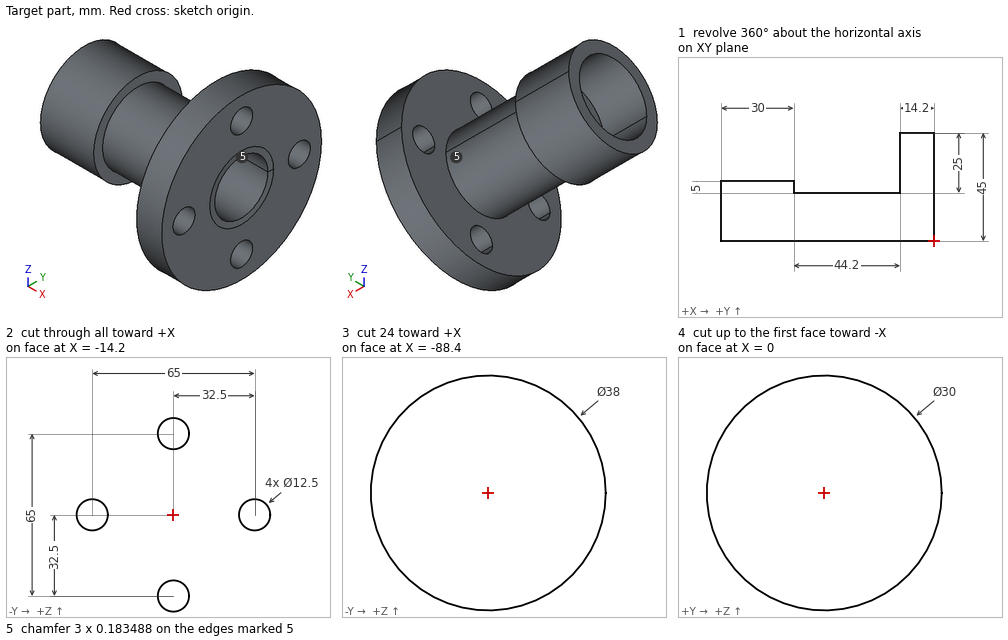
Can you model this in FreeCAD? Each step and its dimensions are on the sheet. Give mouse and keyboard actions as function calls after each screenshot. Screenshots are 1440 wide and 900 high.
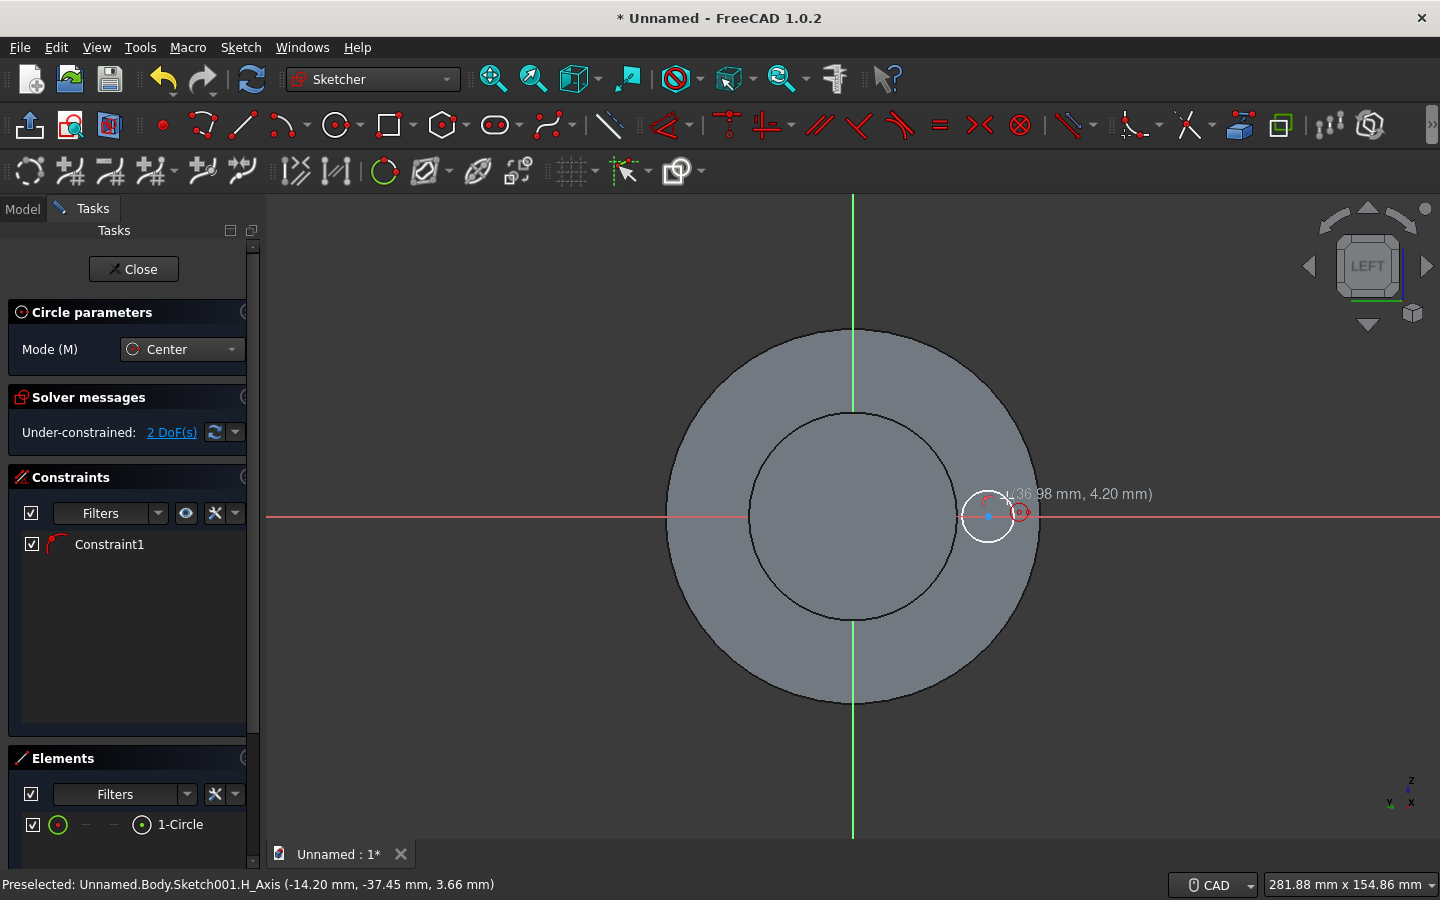
click(853, 652)
click(871, 633)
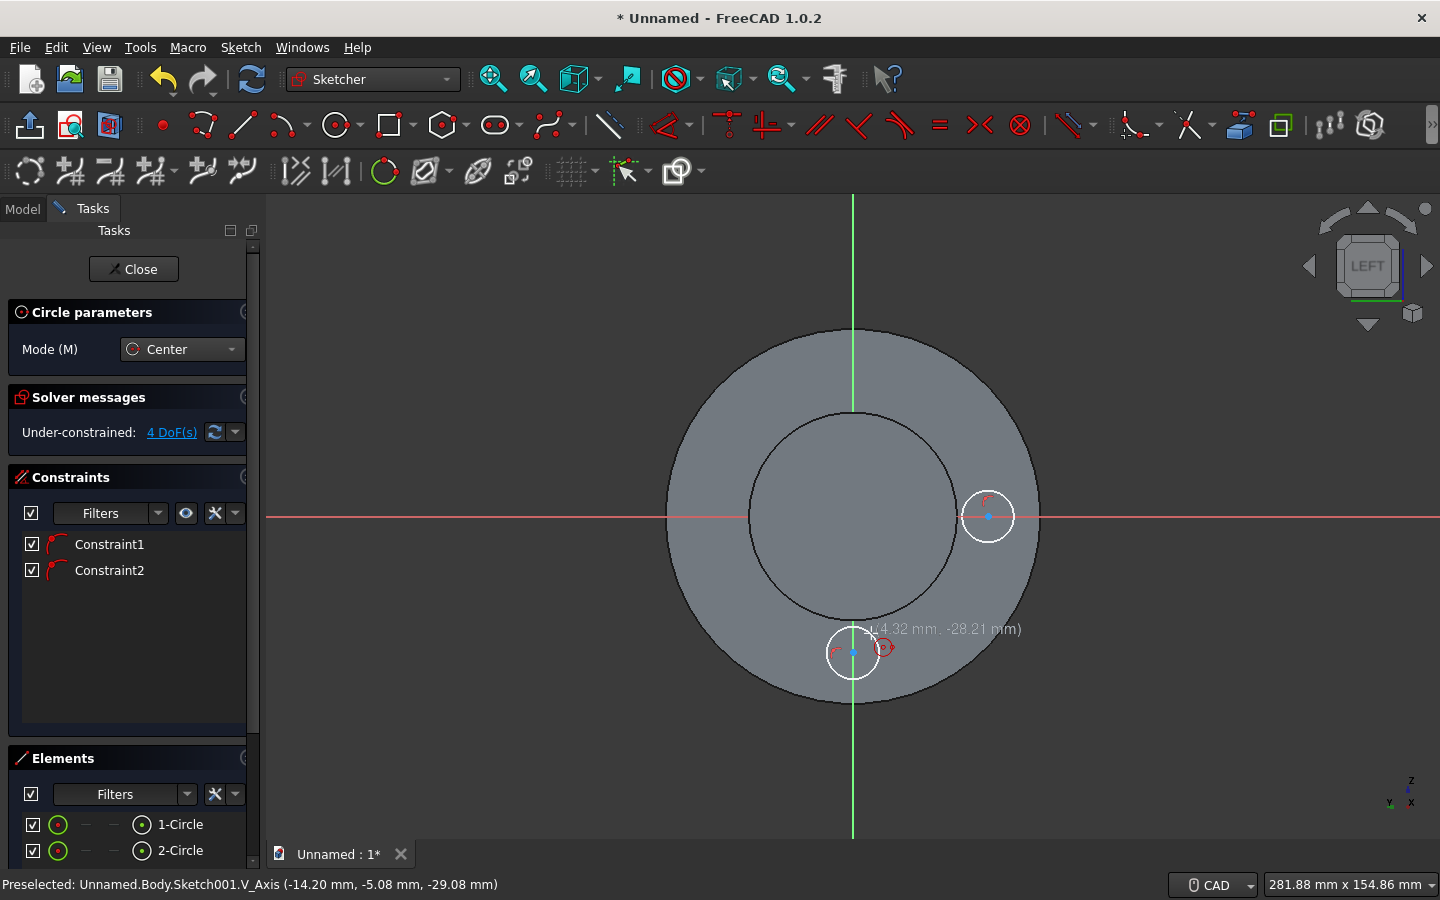
click(718, 516)
click(736, 498)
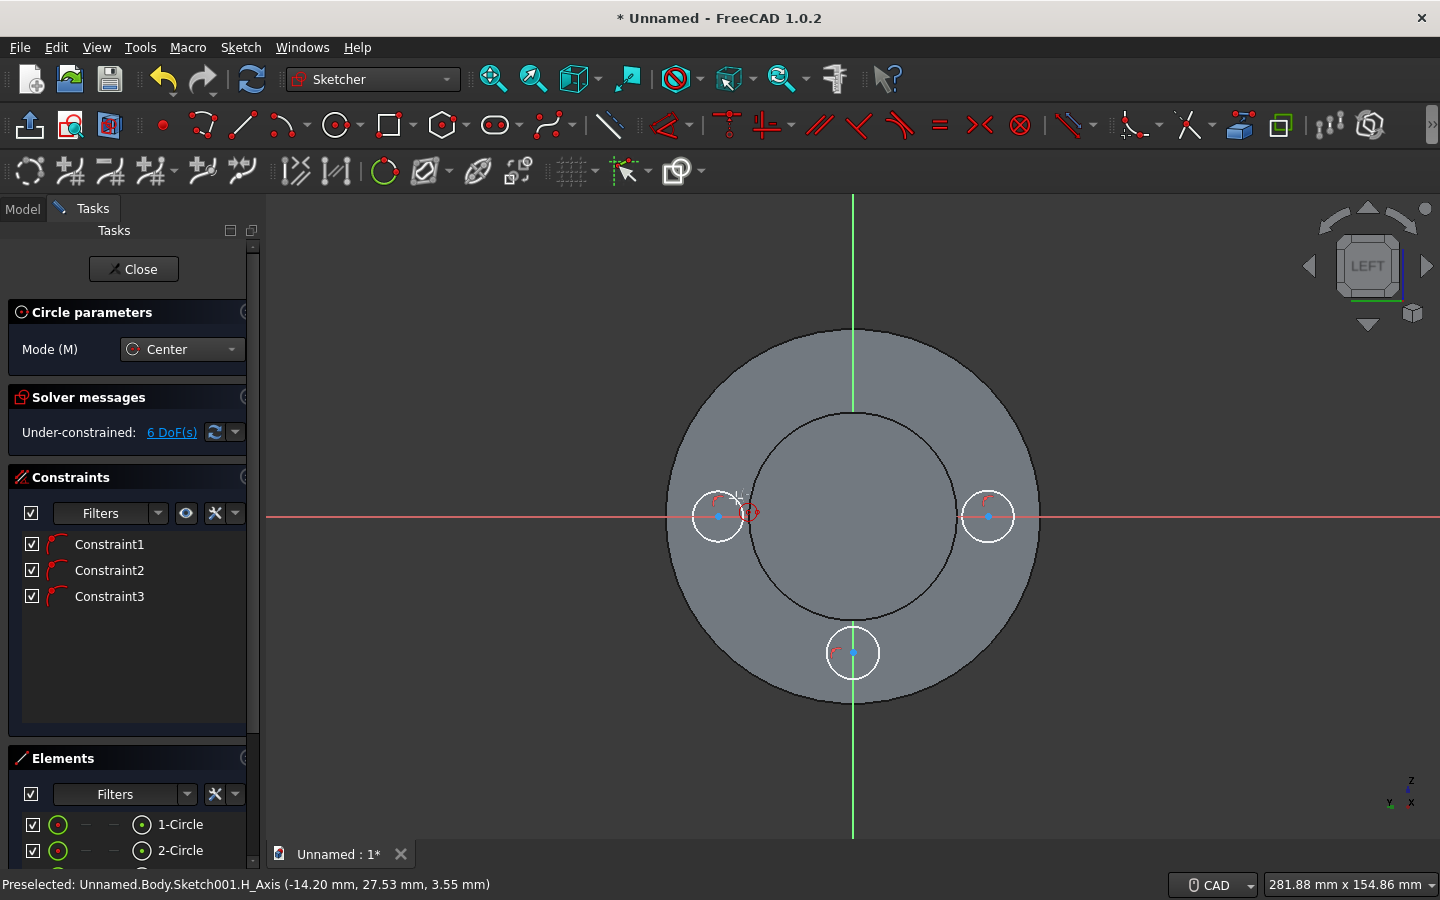
click(853, 381)
click(871, 363)
key(Escape)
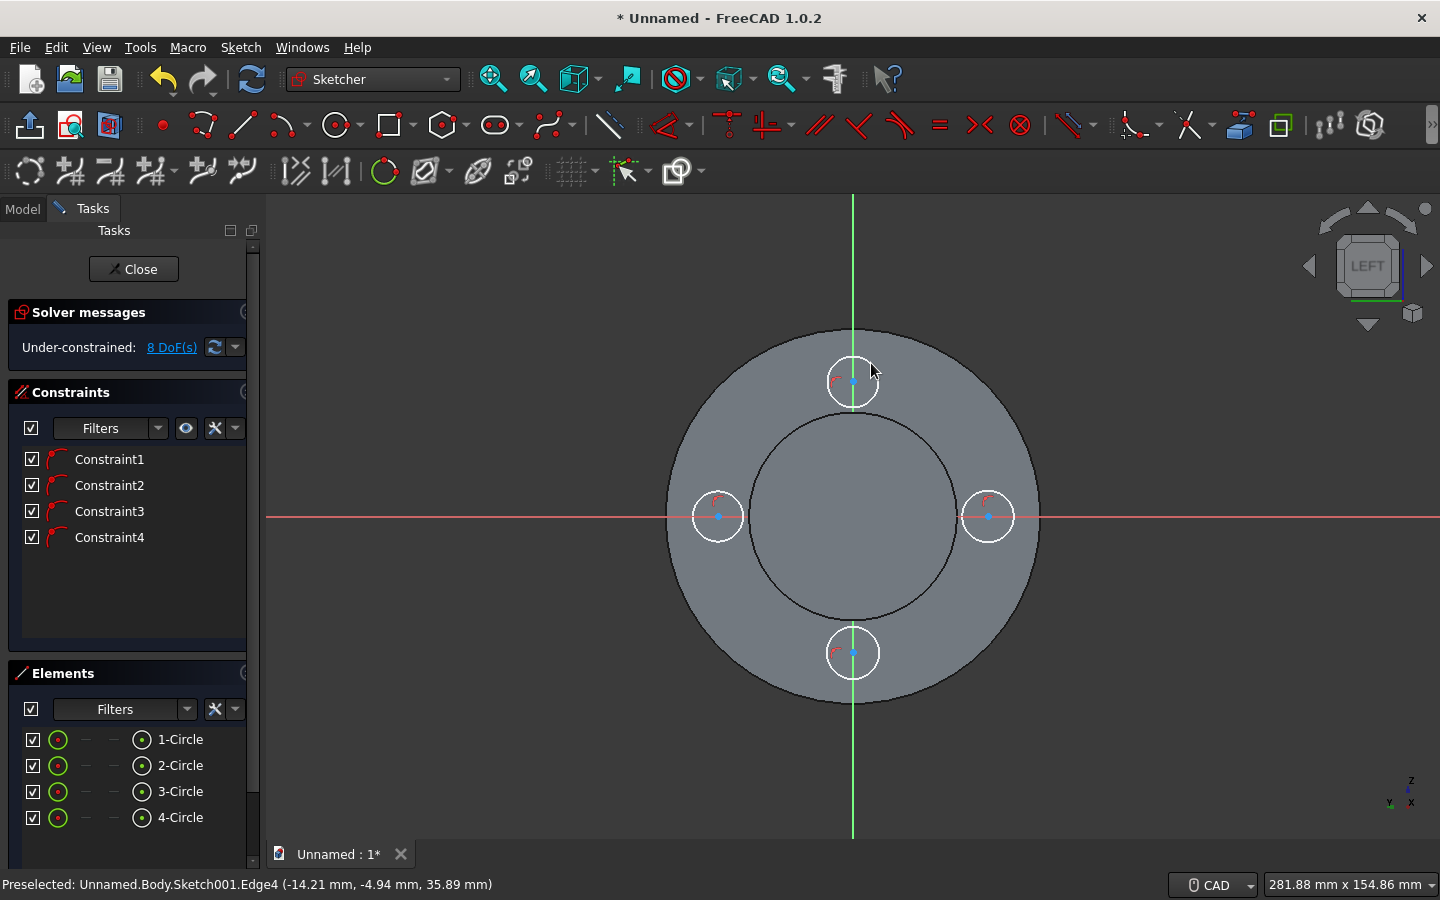
click(1006, 498)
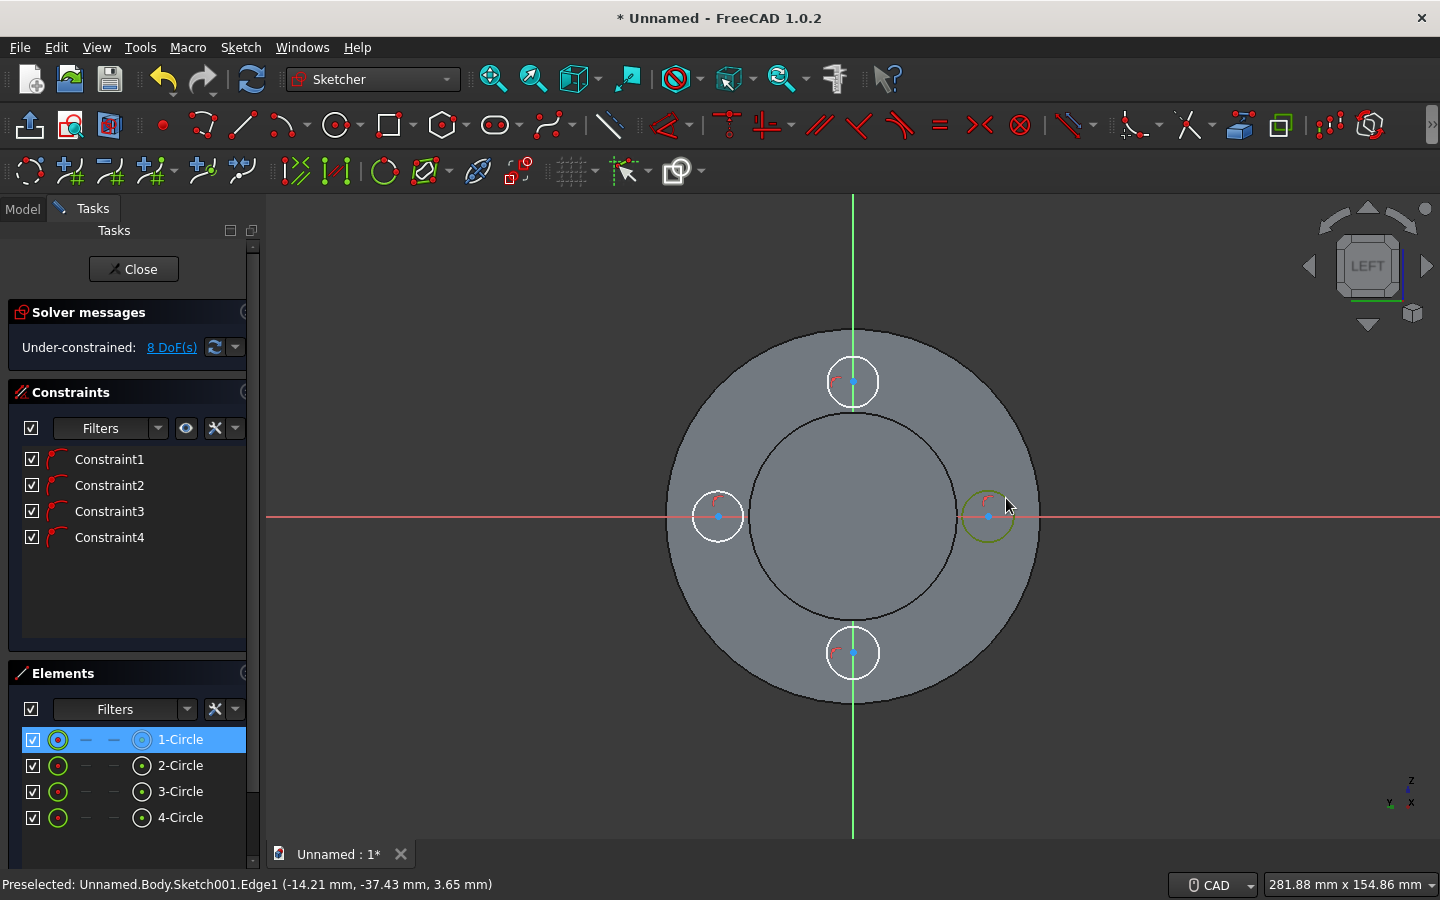
click(871, 634)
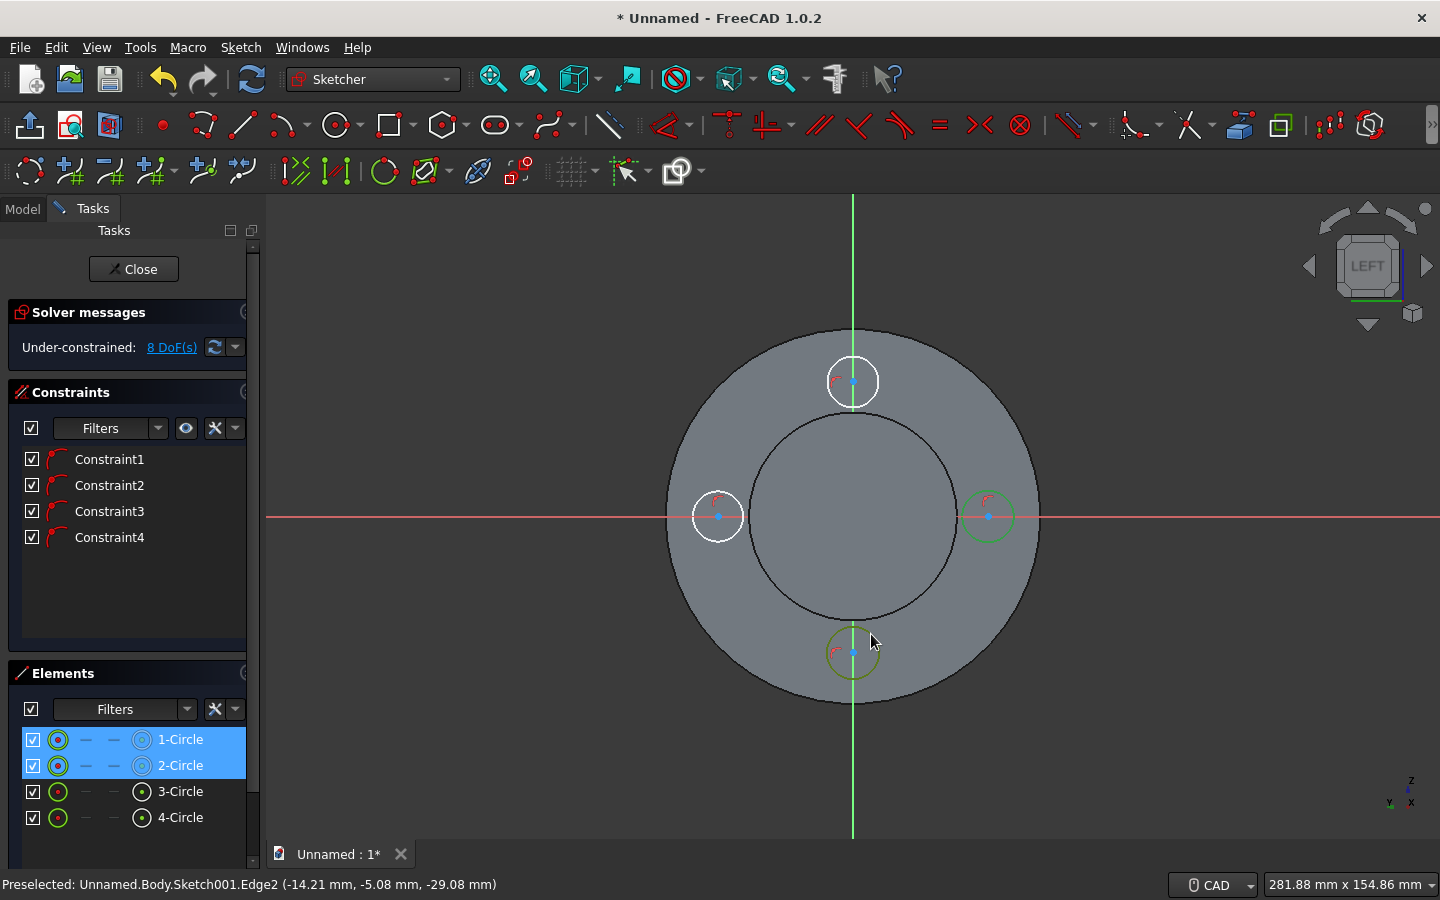
click(736, 499)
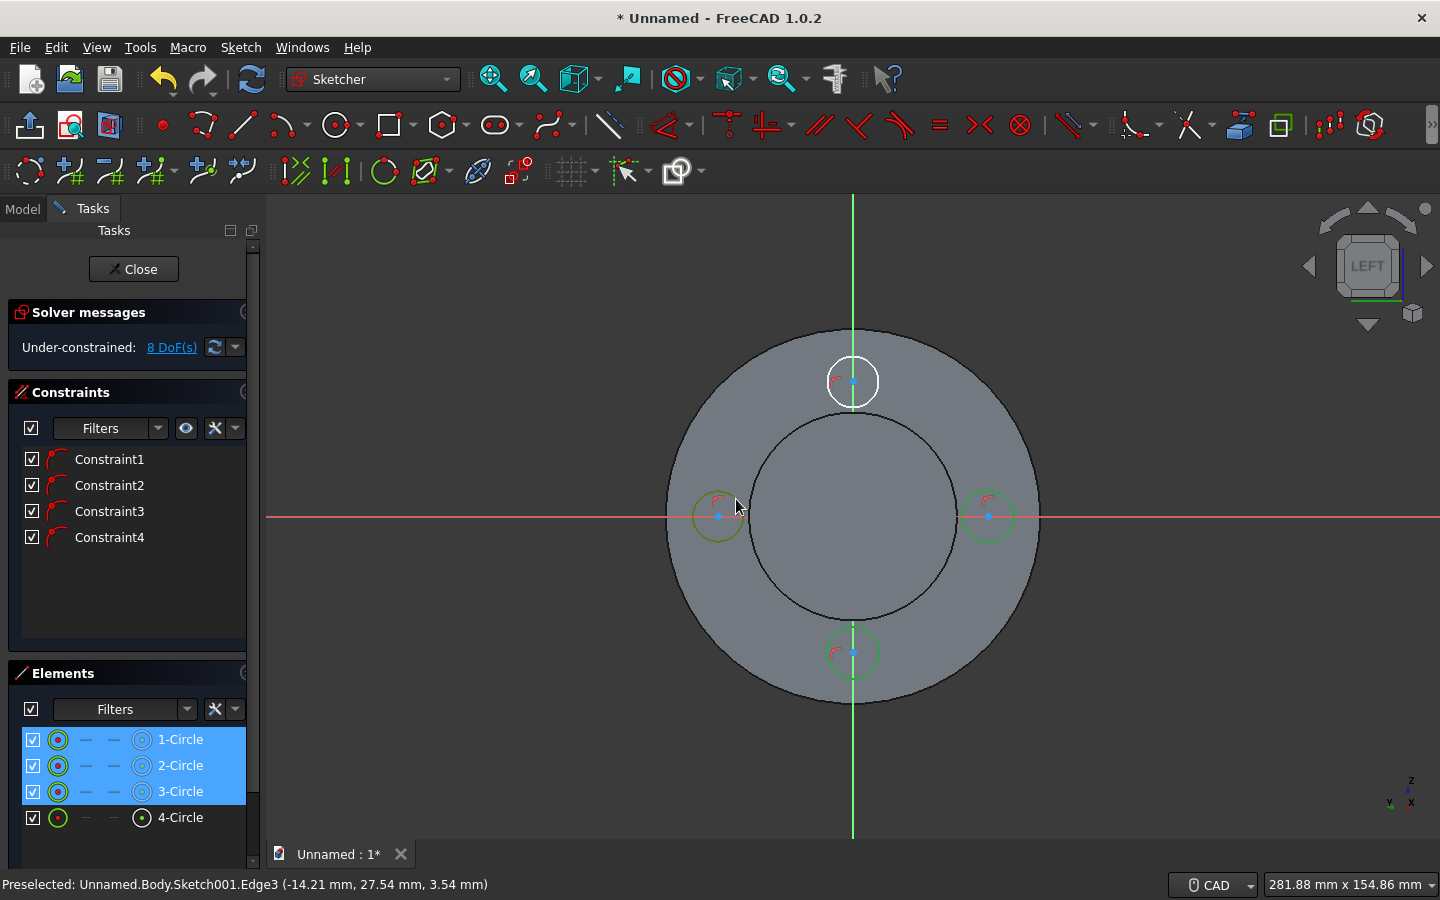
click(871, 364)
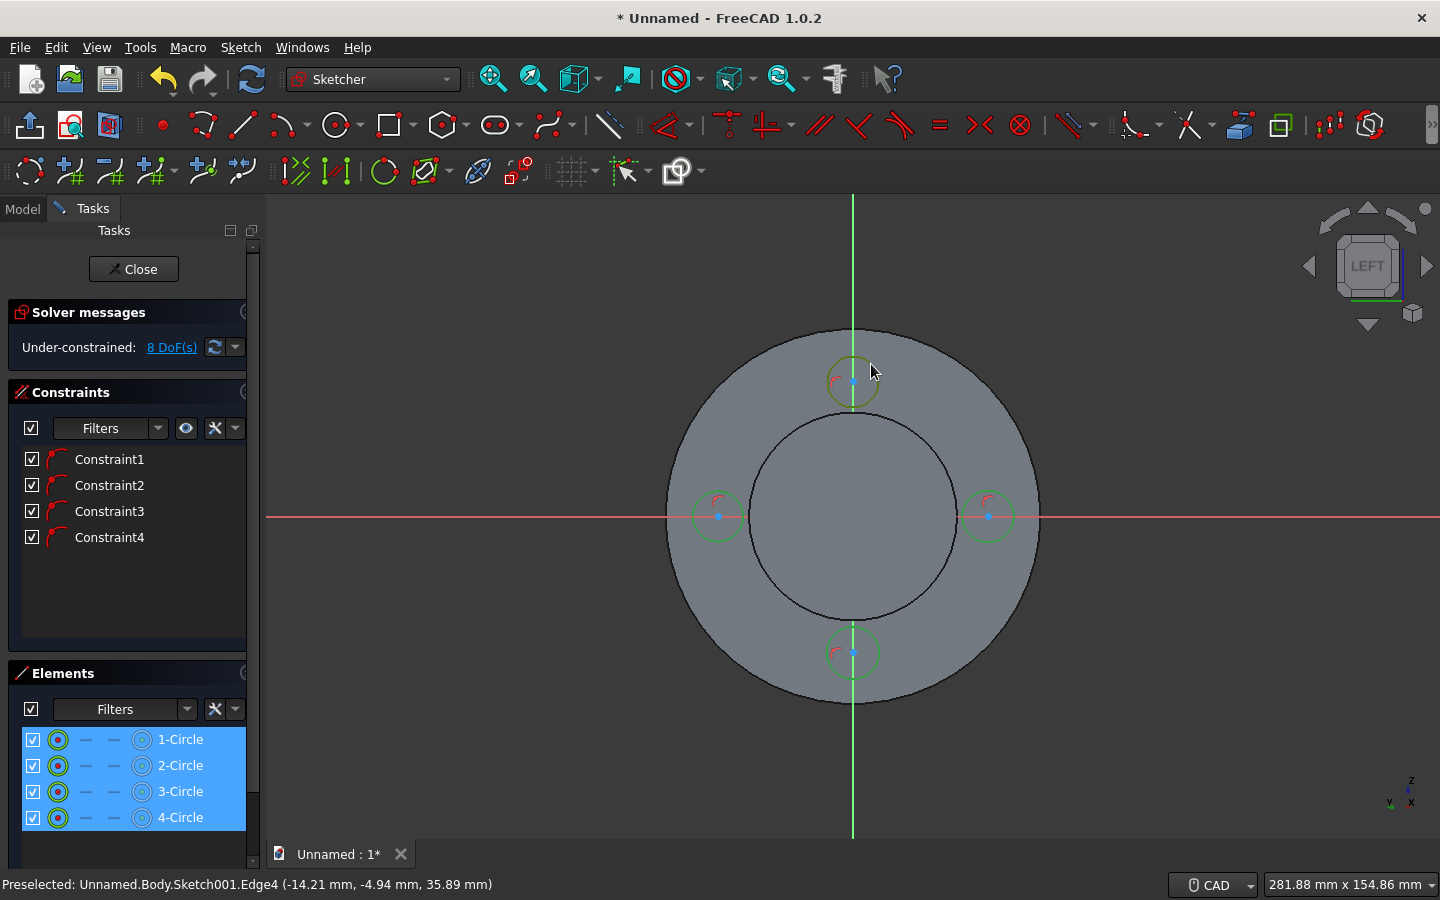
click(940, 126)